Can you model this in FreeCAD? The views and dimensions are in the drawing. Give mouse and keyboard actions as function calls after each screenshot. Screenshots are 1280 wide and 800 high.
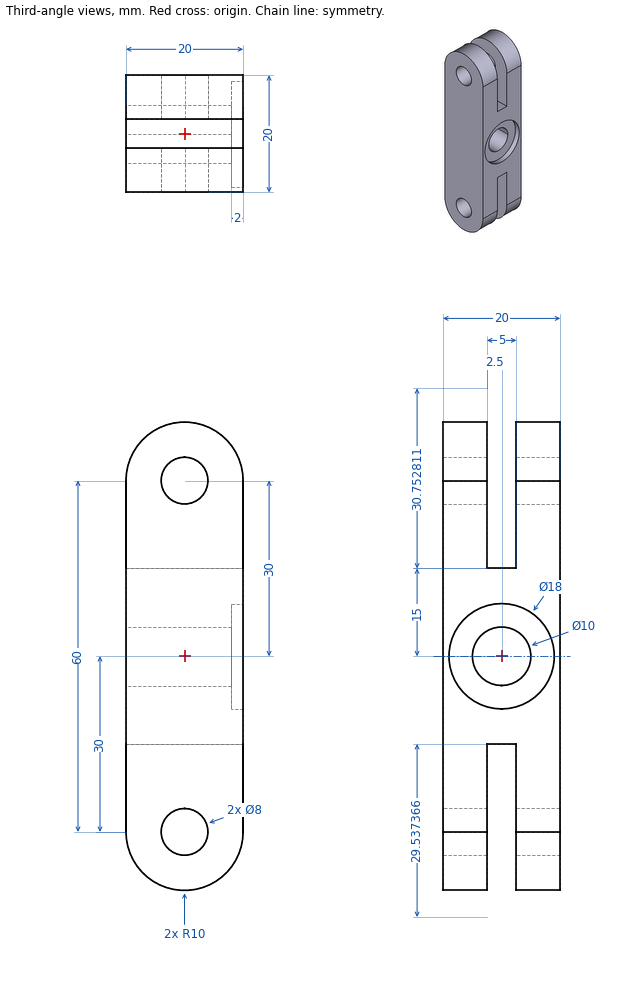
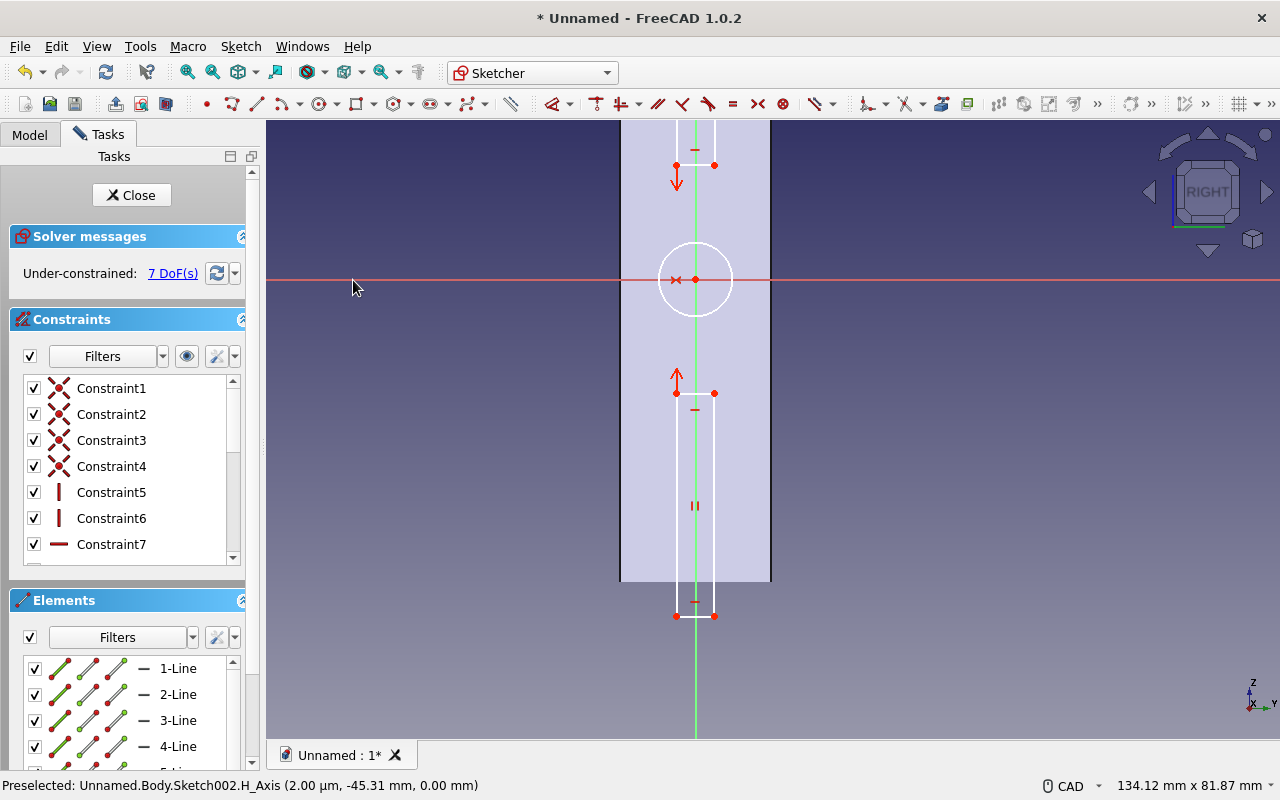
click(552, 104)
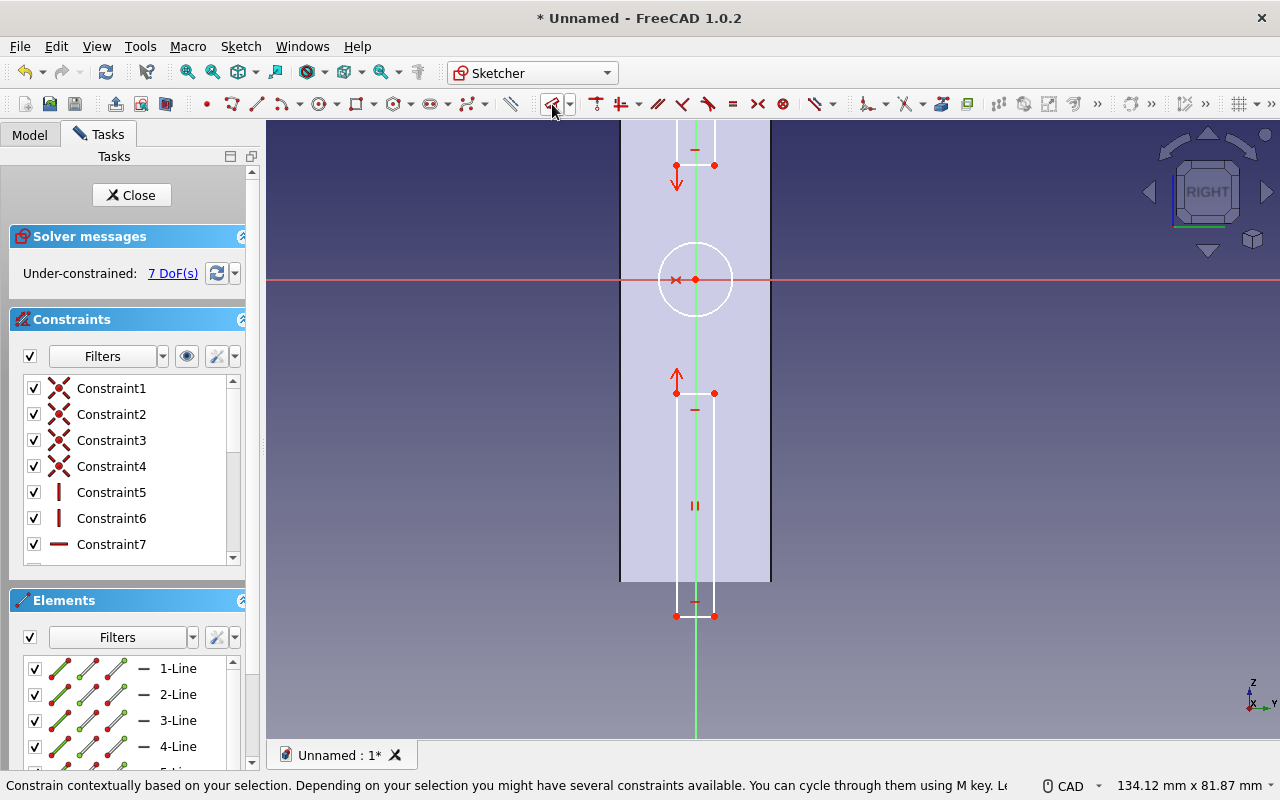
click(721, 253)
click(743, 230)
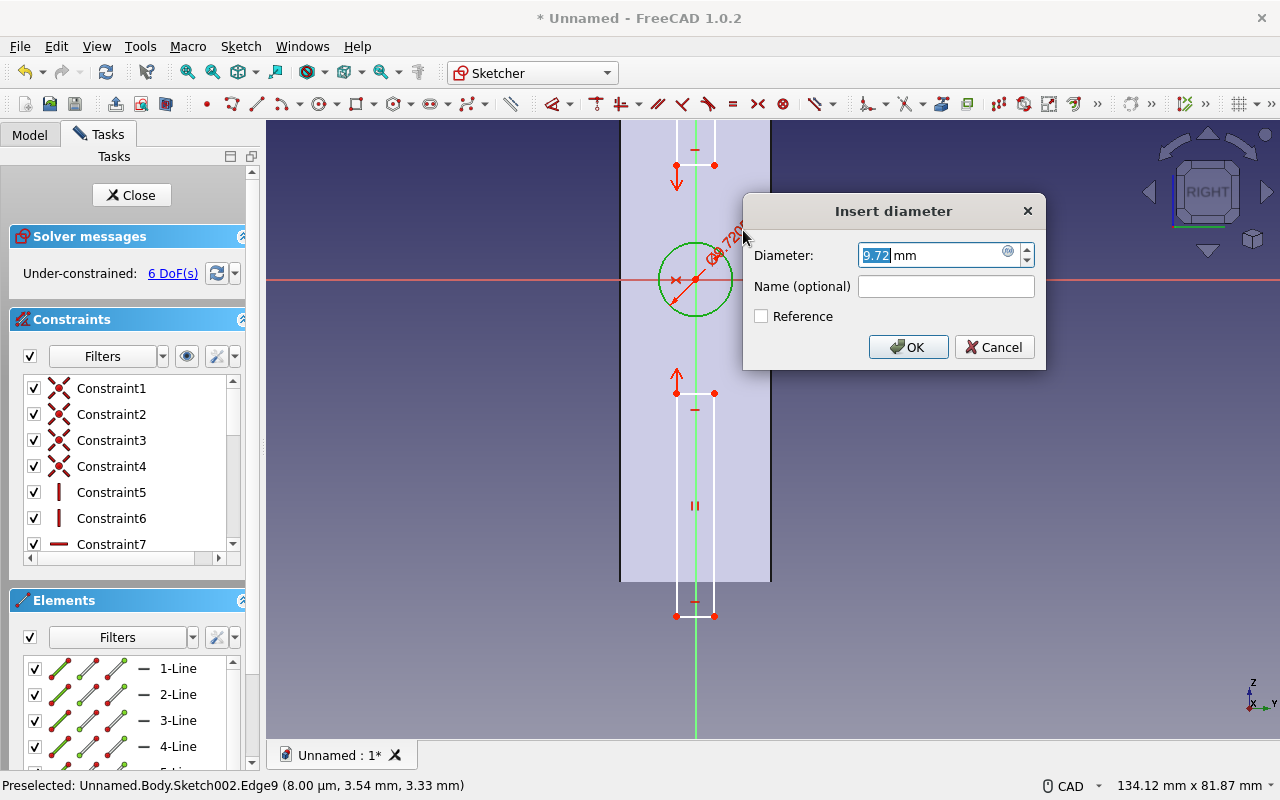
text(10)
key(Return)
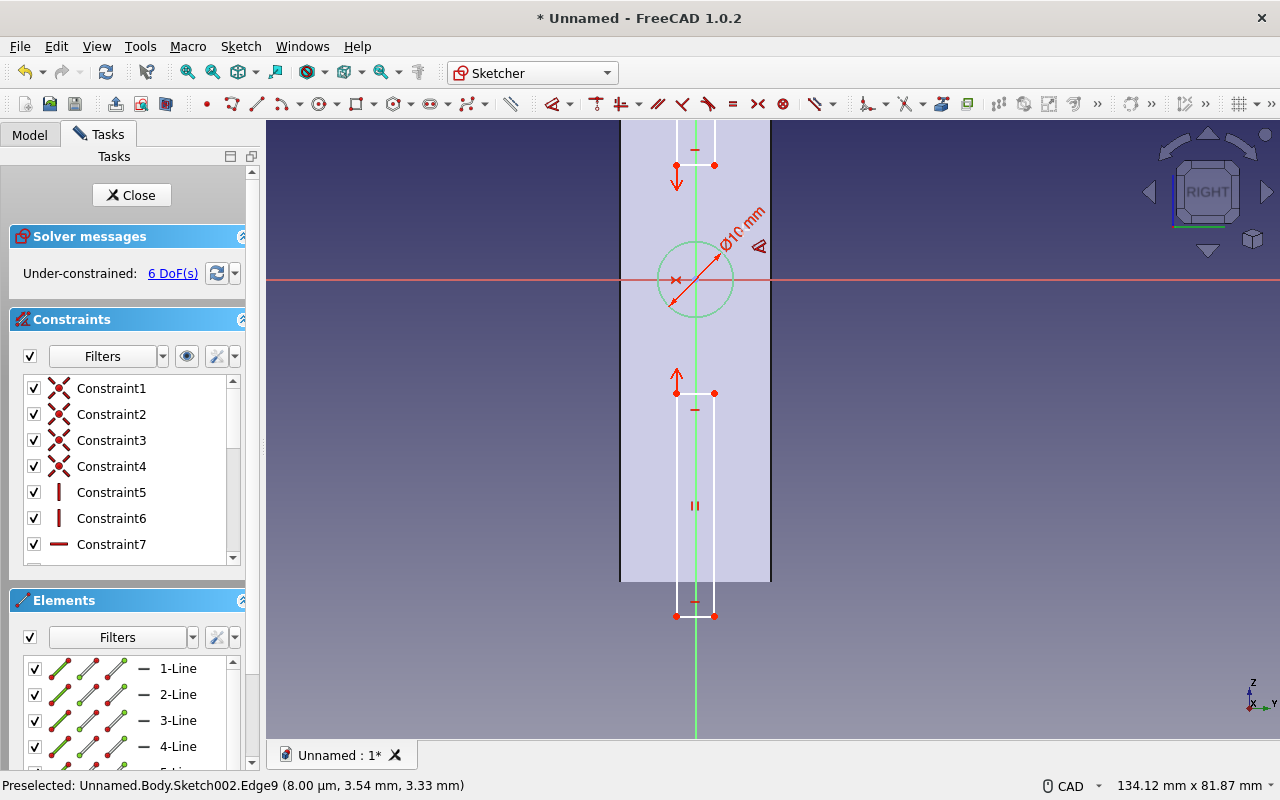
click(692, 165)
click(682, 199)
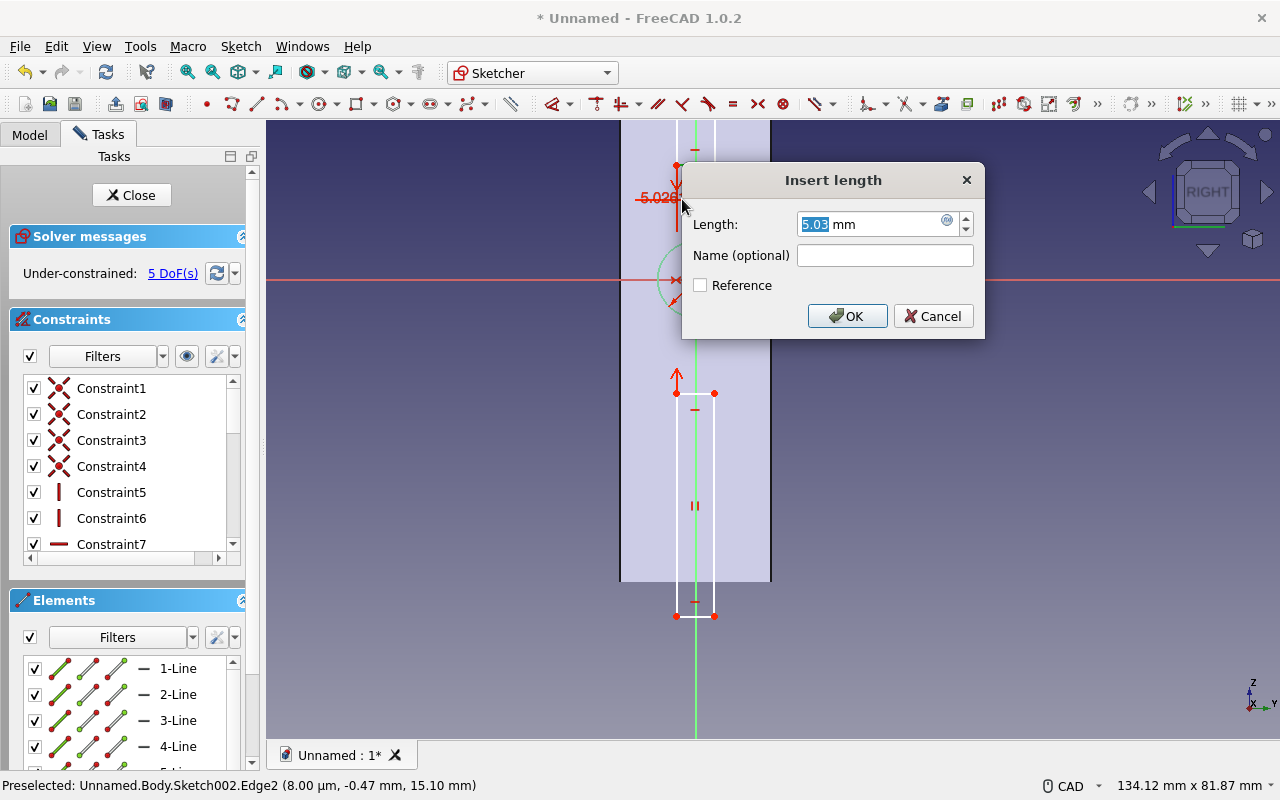
text(5)
key(Return)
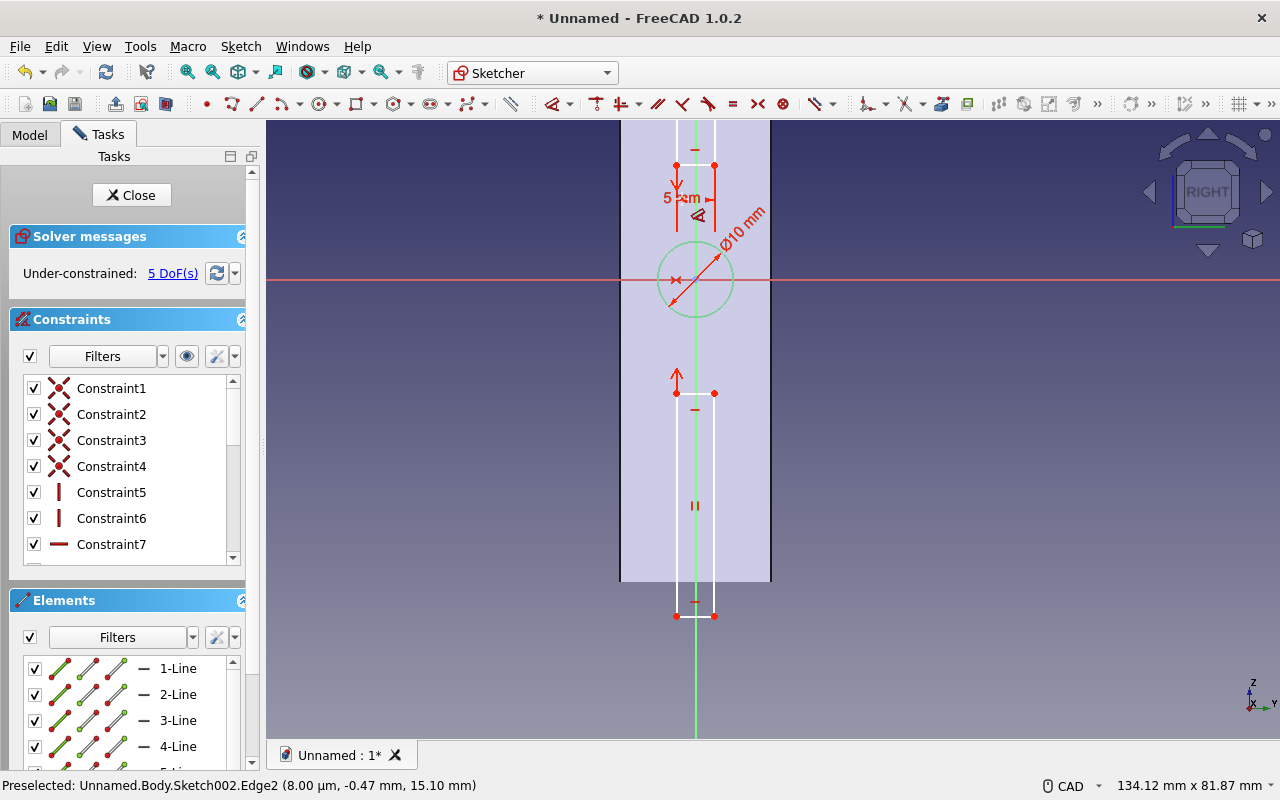
click(692, 617)
click(682, 651)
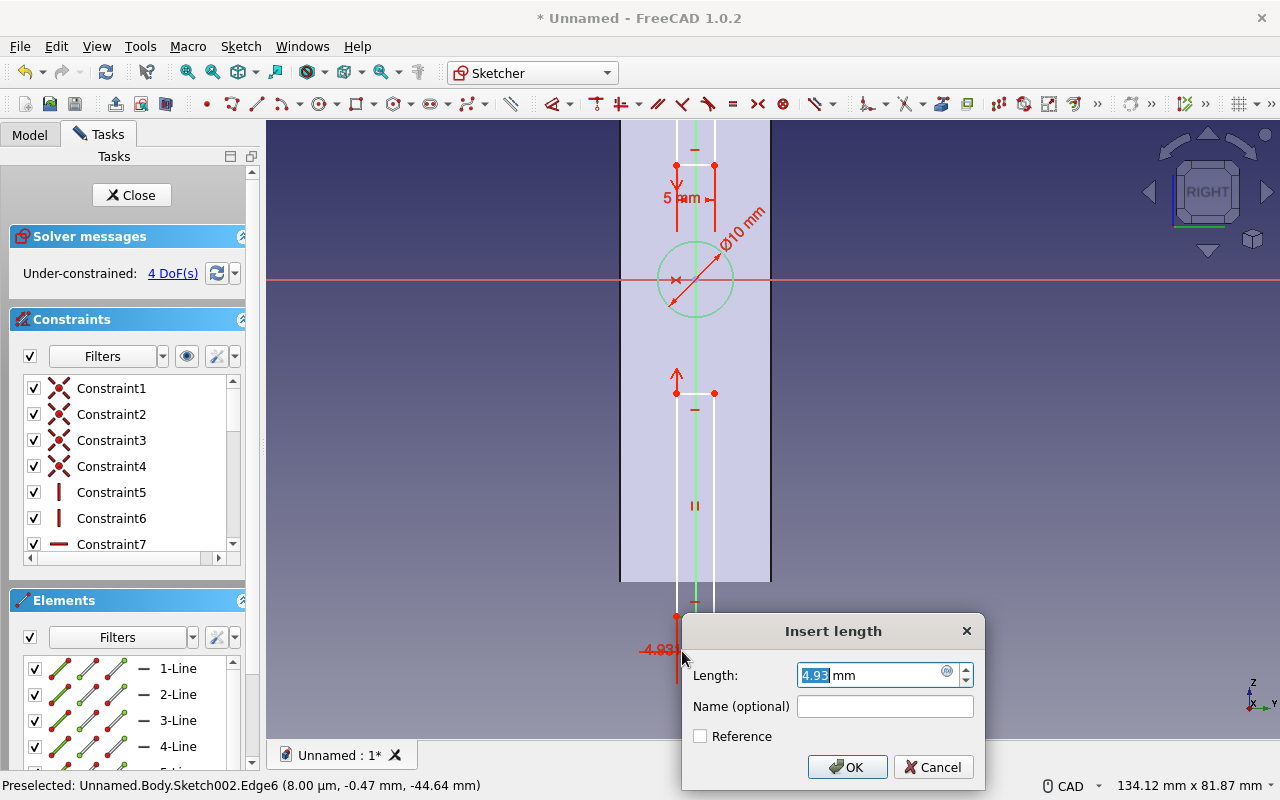
text(5)
key(Return)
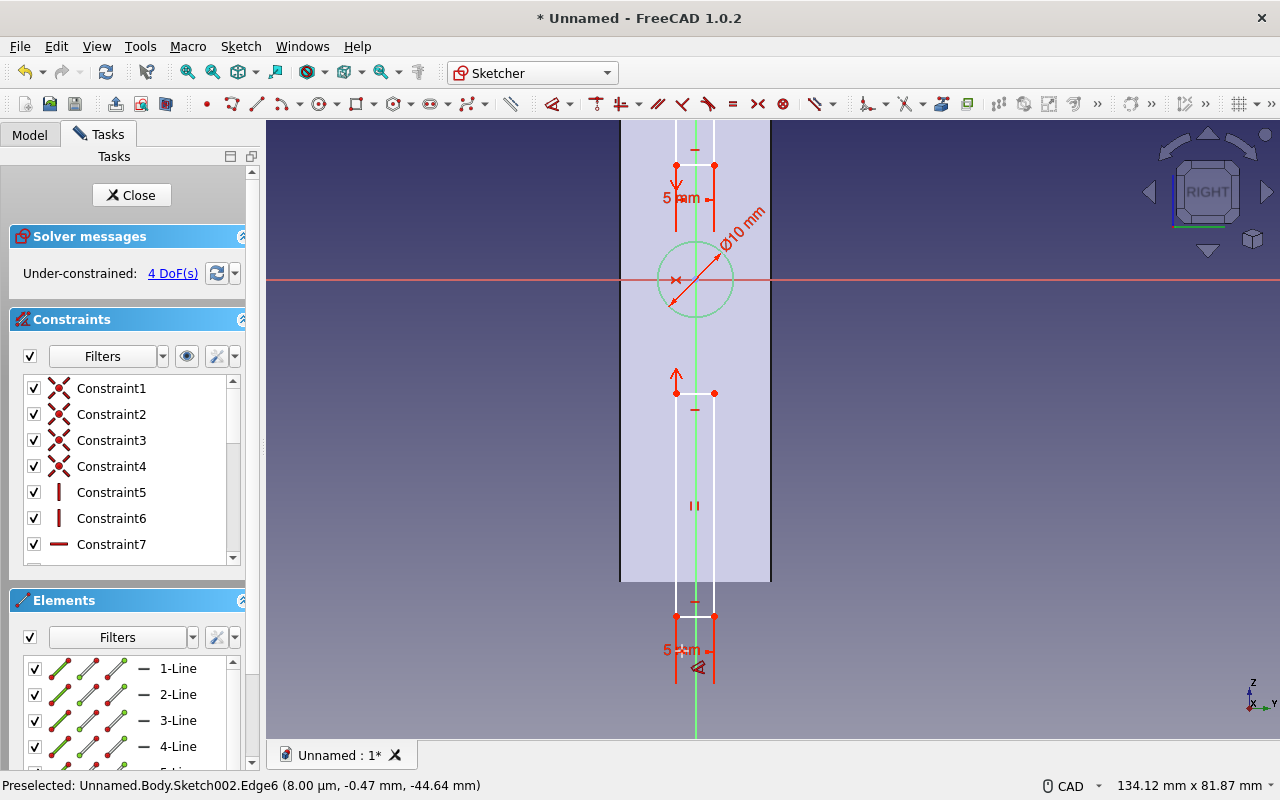
click(676, 165)
click(642, 222)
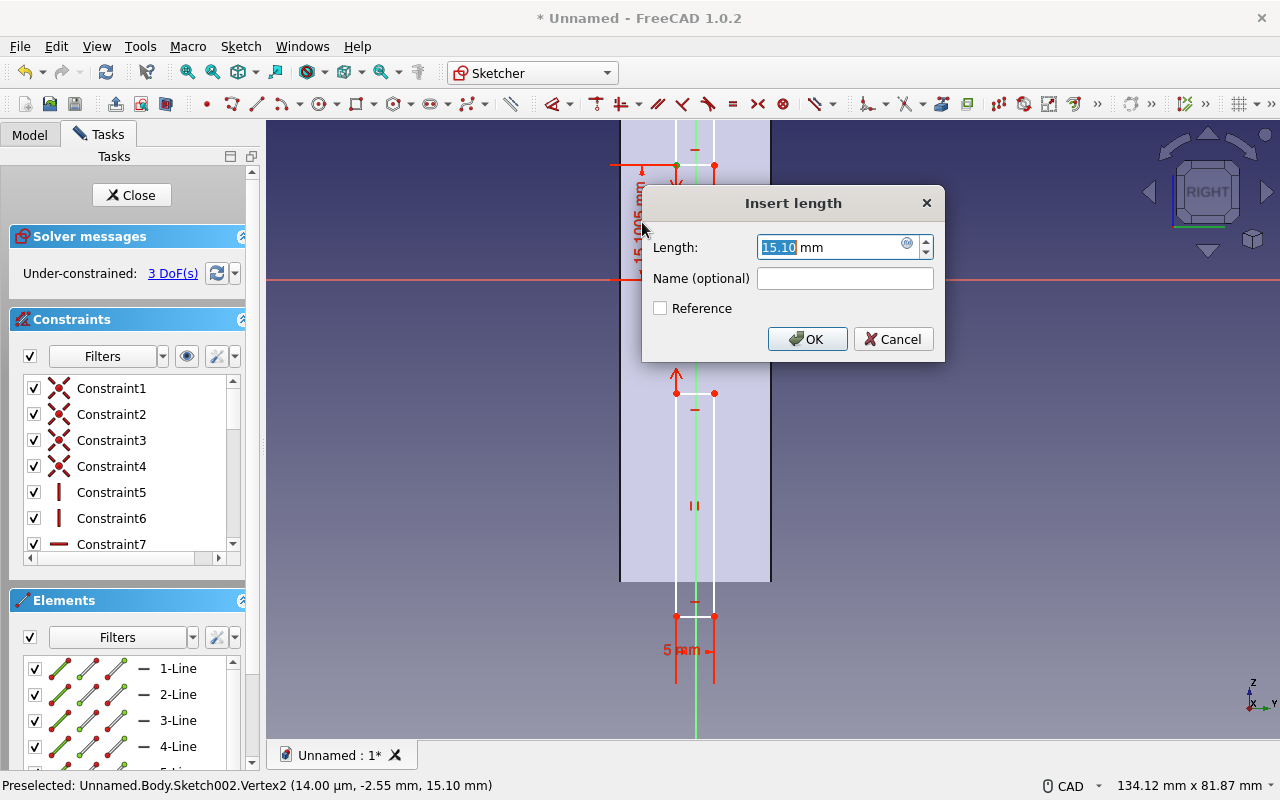
text(15)
key(Return)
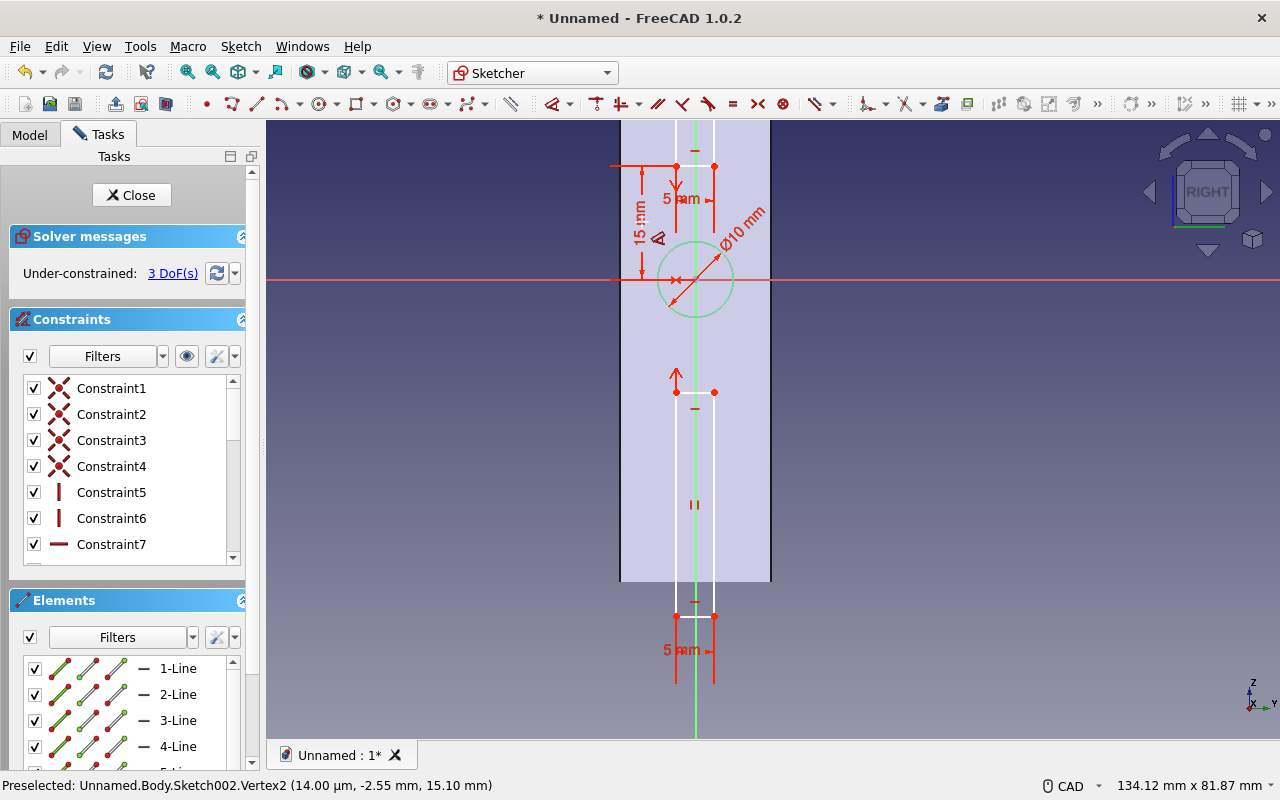
scroll(715, 618, down, 3)